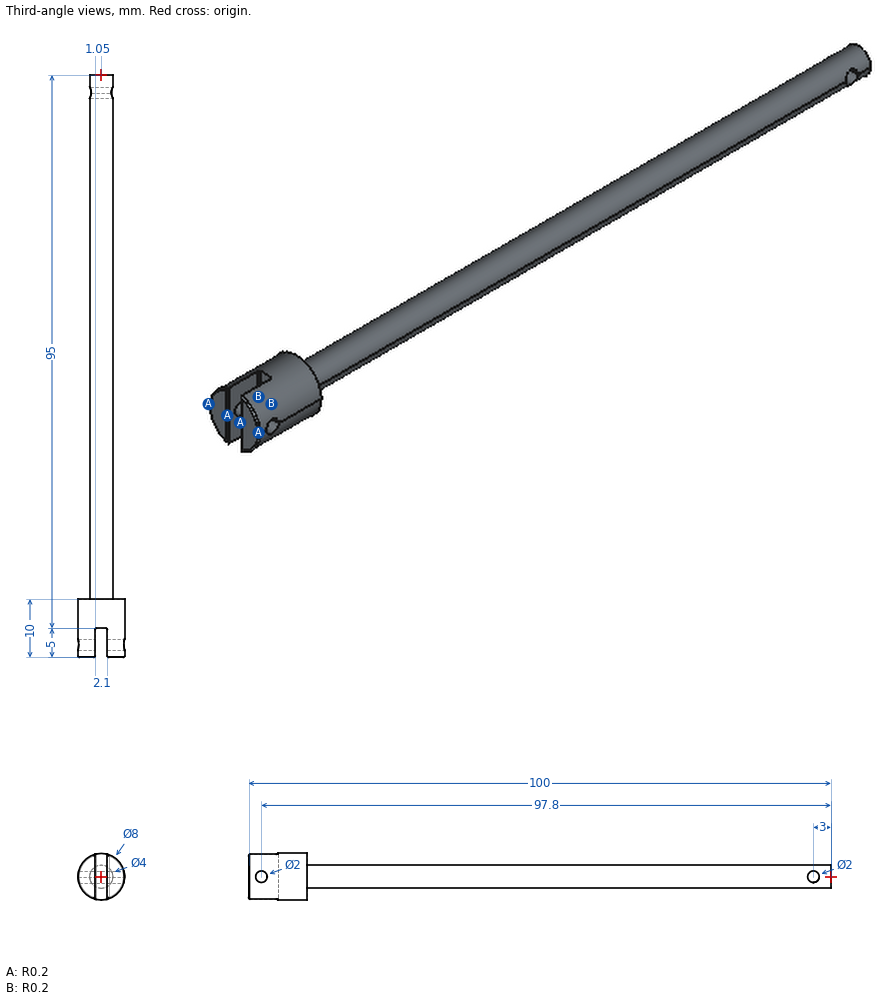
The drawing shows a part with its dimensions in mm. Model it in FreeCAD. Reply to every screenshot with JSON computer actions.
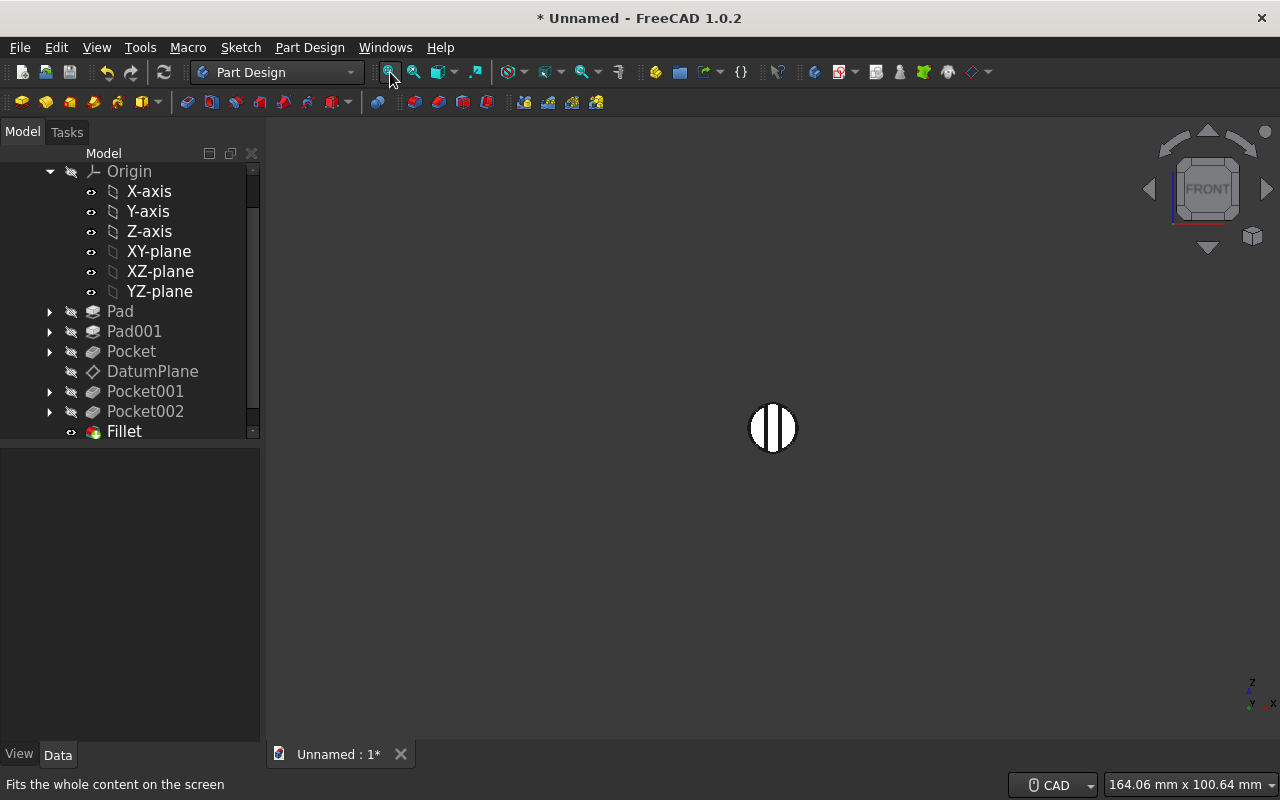
{"action": "left_click", "coordinate": [390, 72]}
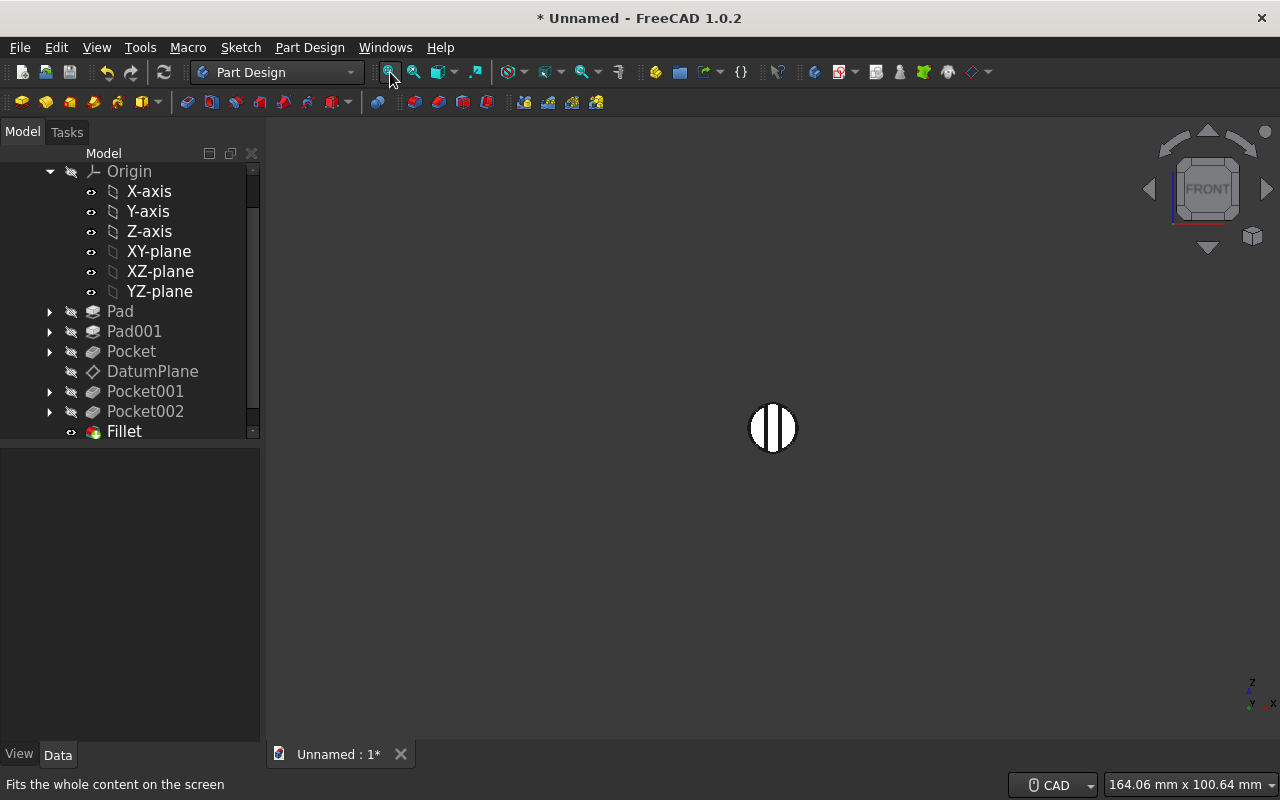
{"action": "key", "text": "3"}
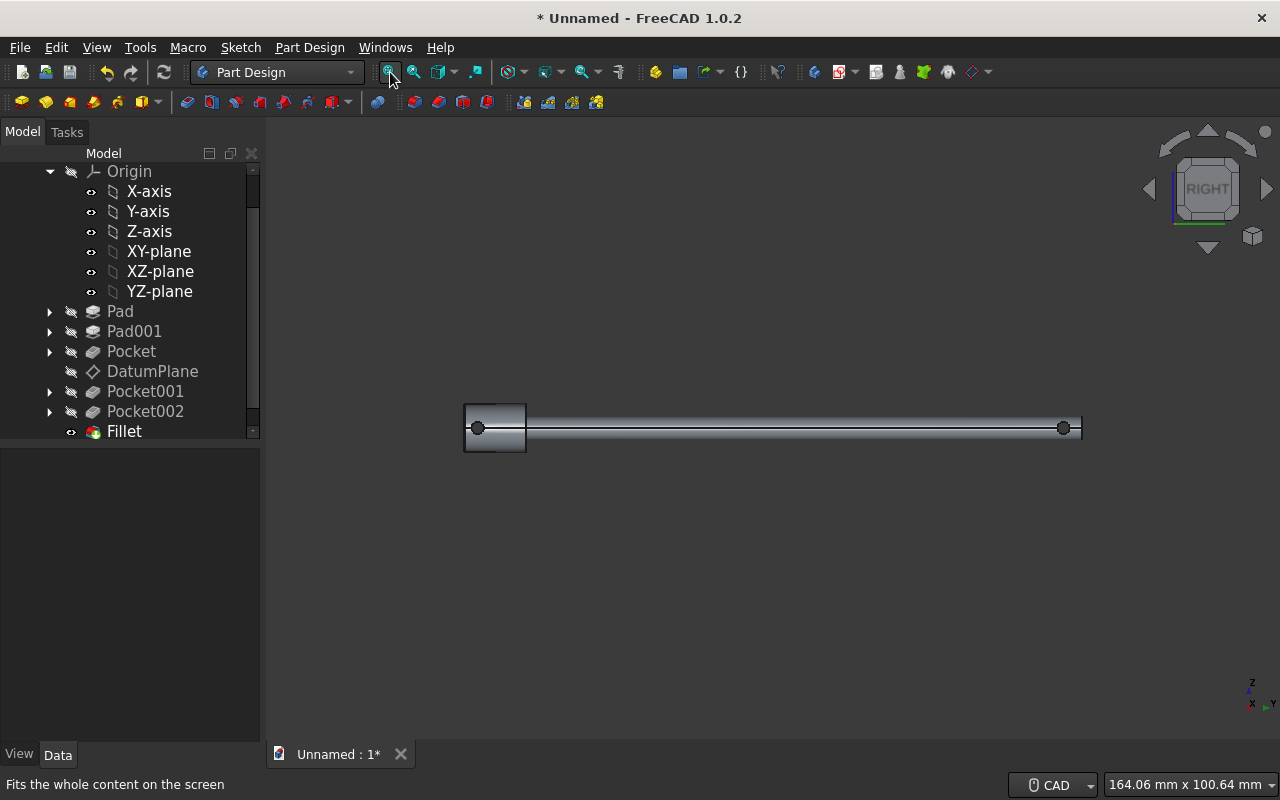
{"action": "key", "text": "5"}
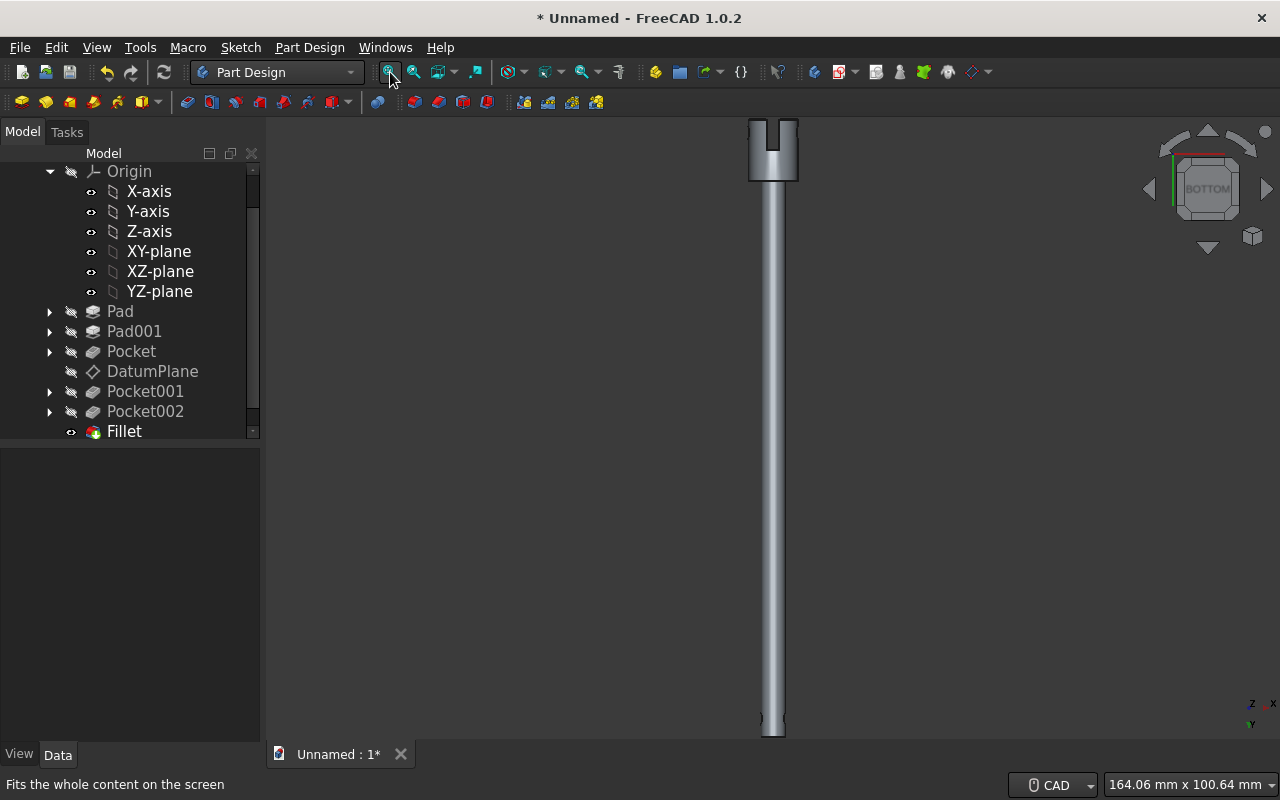
{"action": "key", "text": "4"}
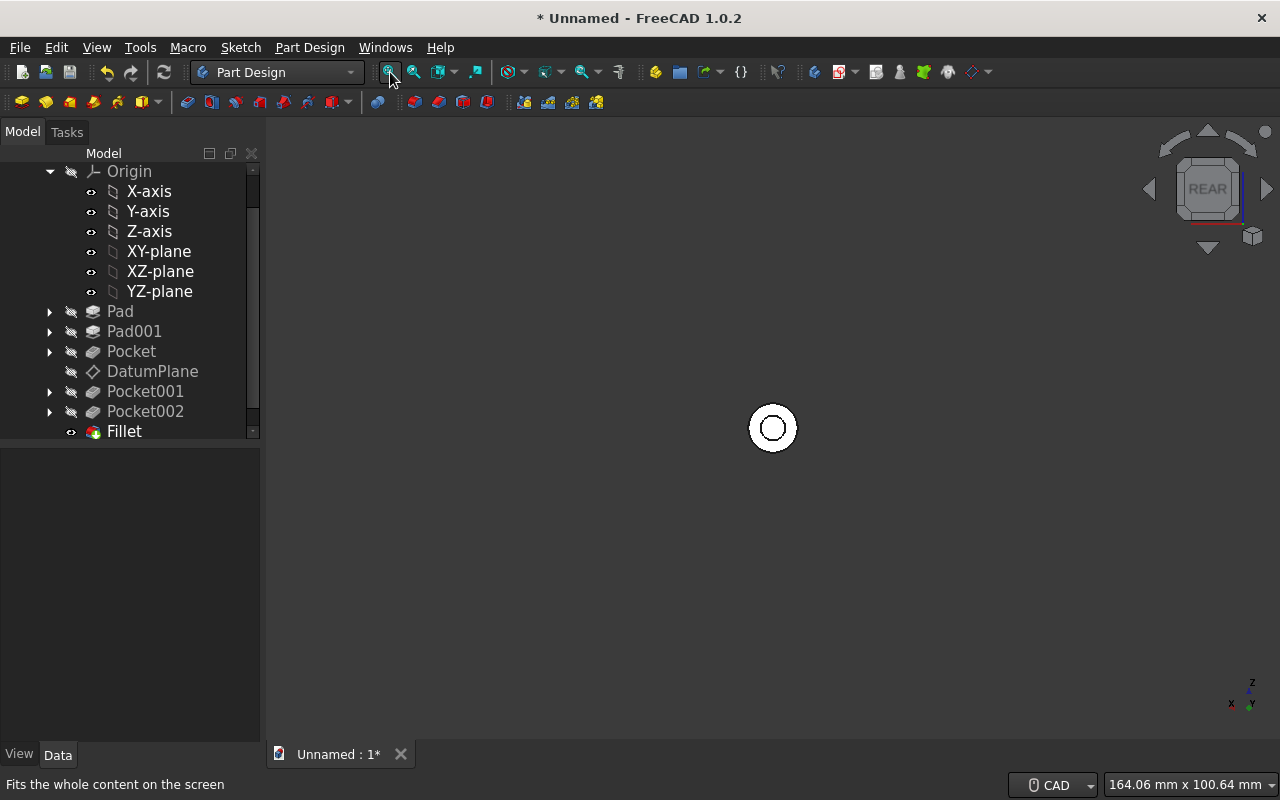
{"action": "left_click", "coordinate": [390, 72]}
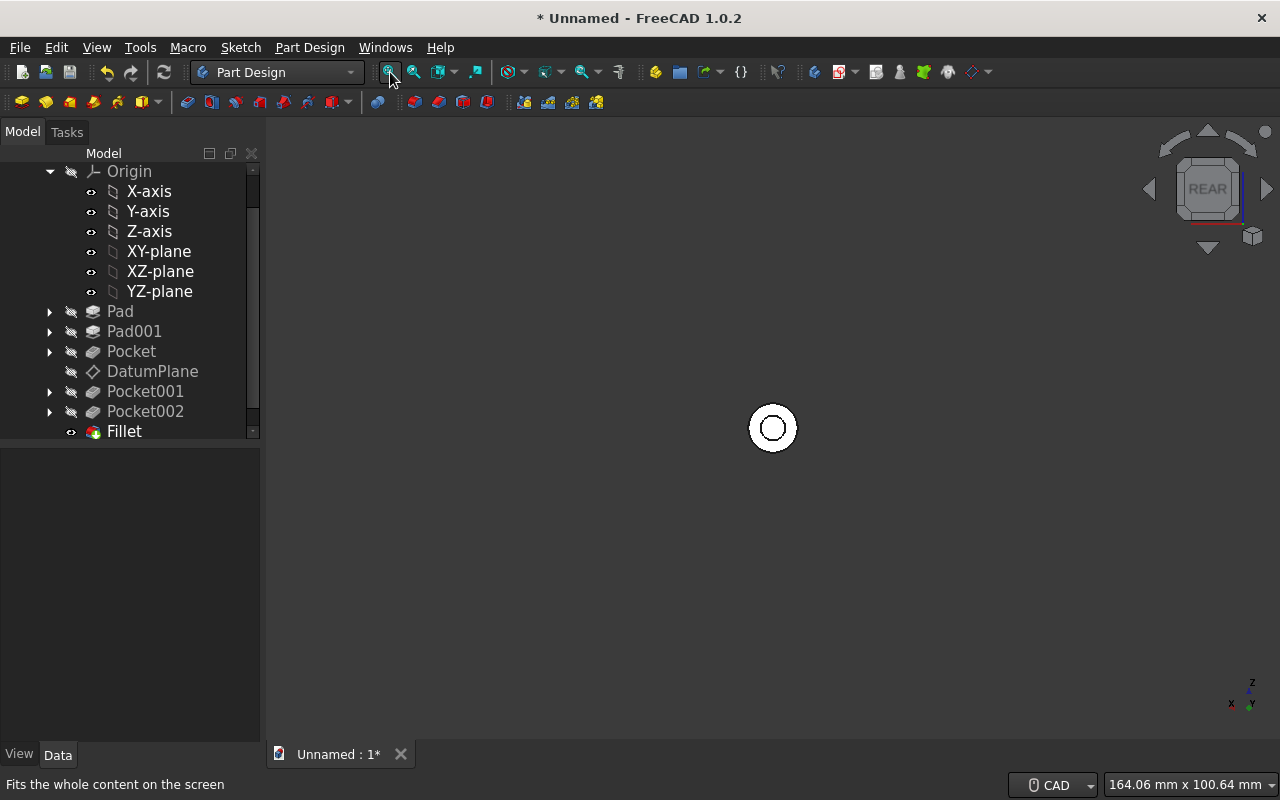
{"action": "key", "text": "6"}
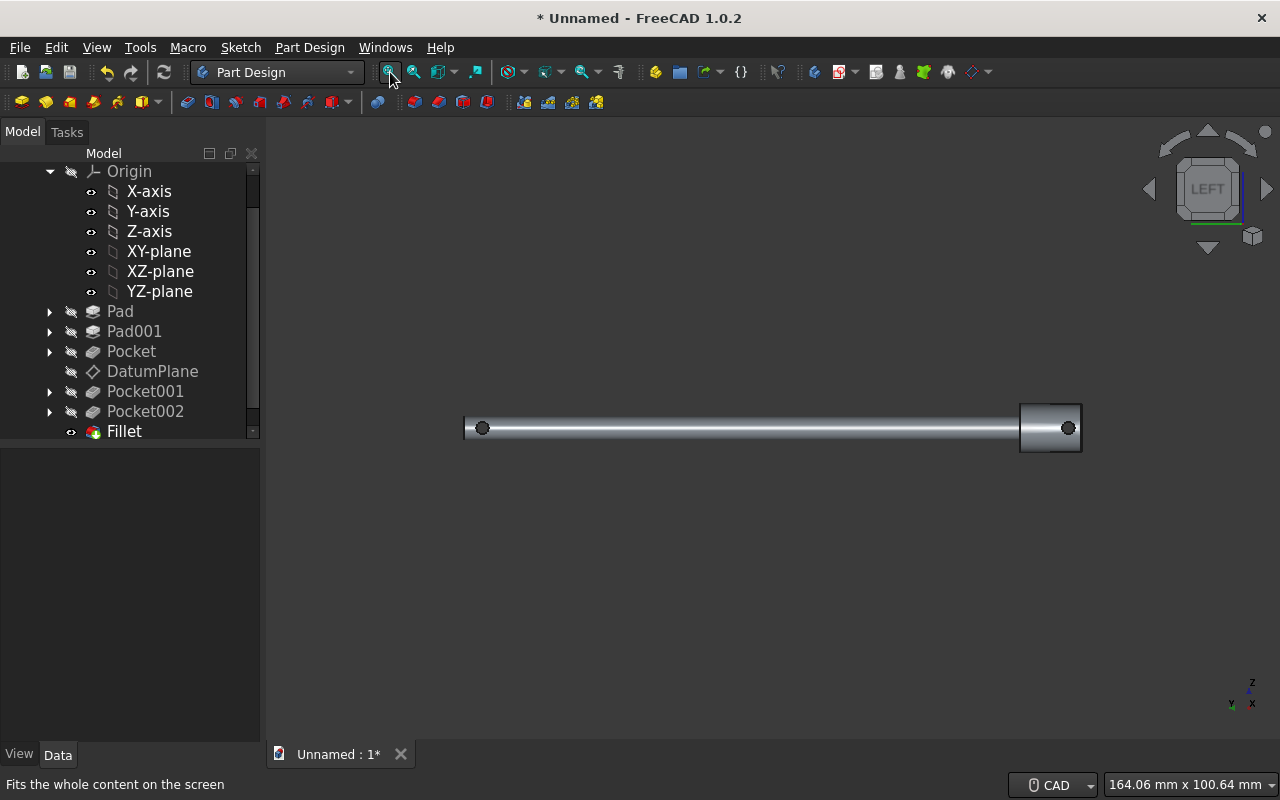
{"action": "key", "text": "v 3"}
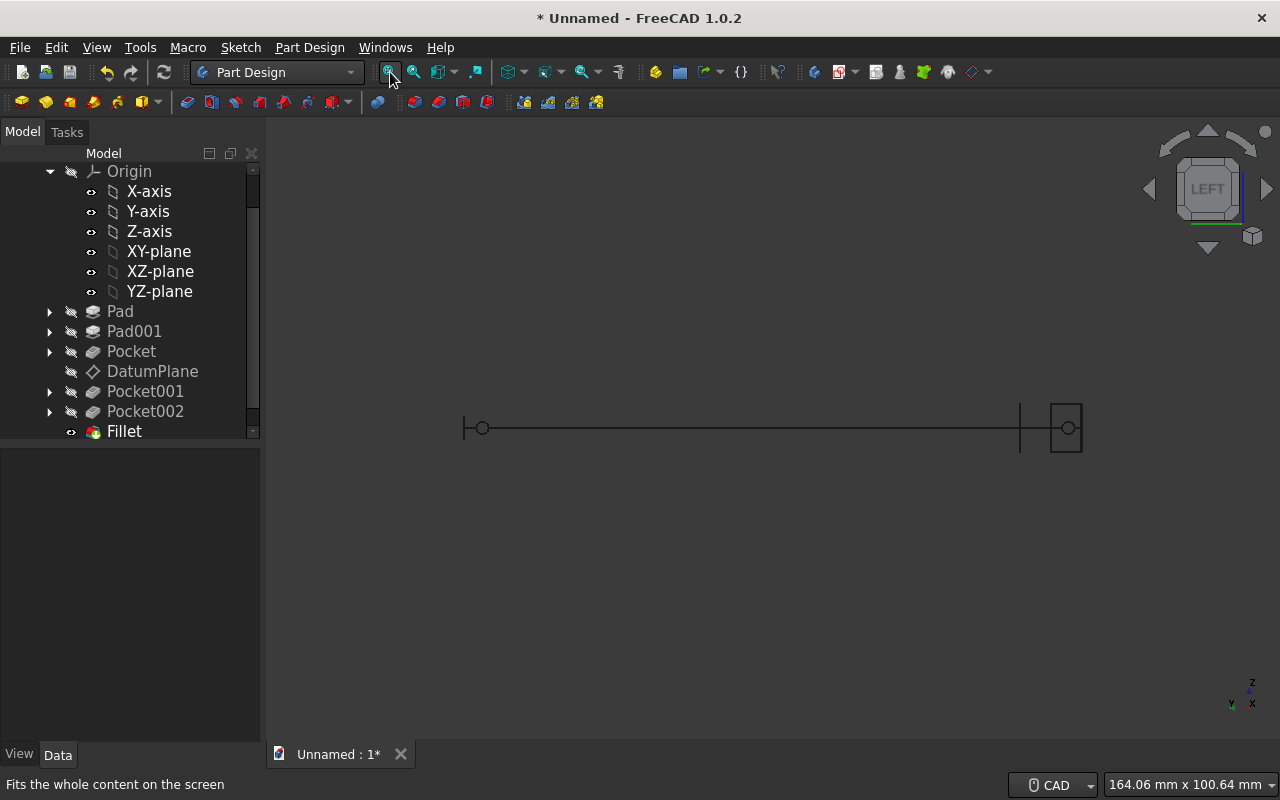
{"action": "key", "text": "0"}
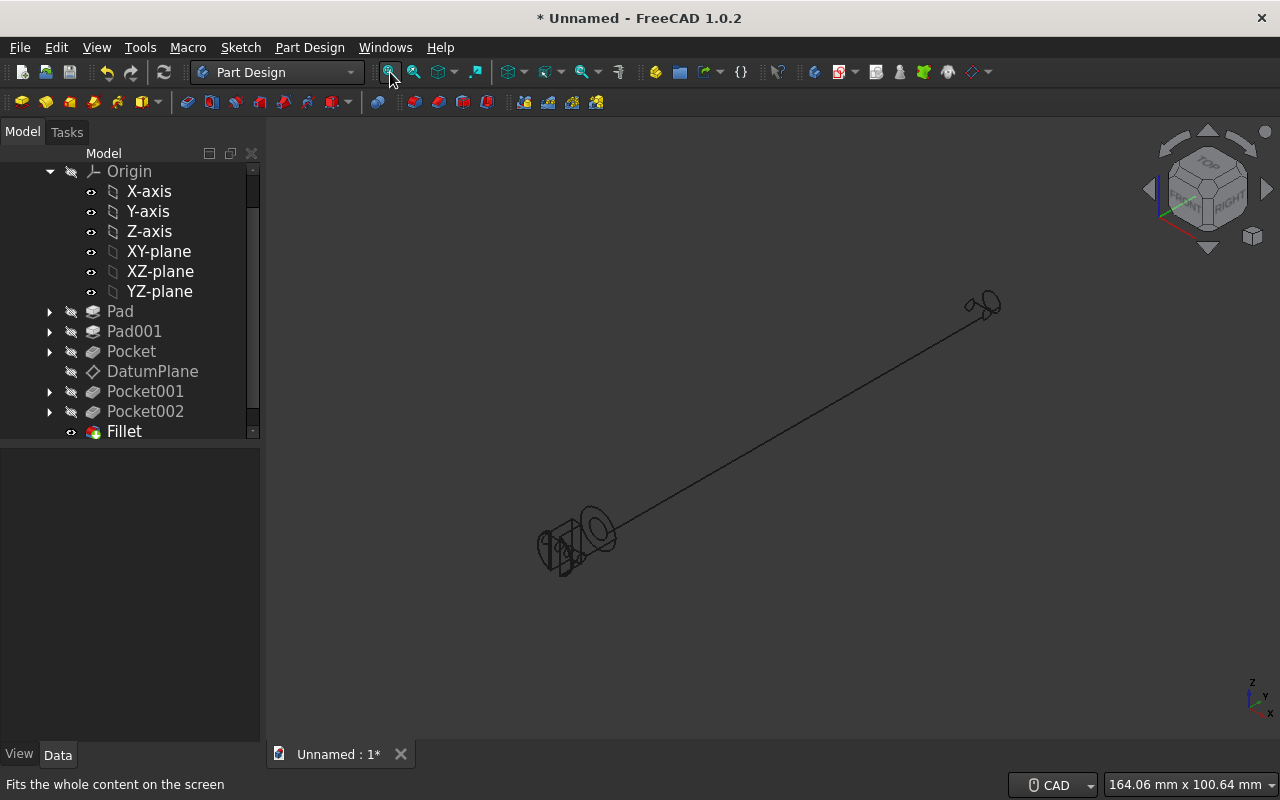
{"action": "left_click", "coordinate": [572, 538]}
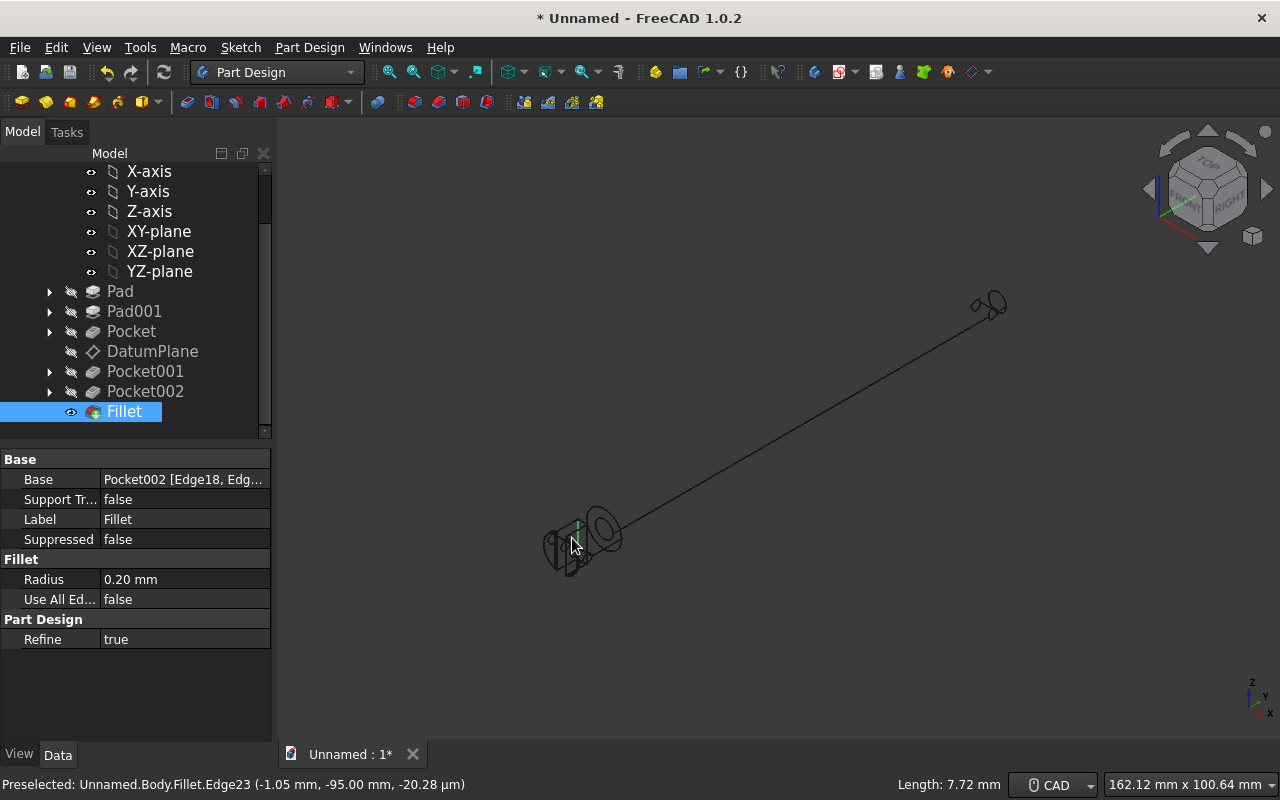
{"action": "left_click", "coordinate": [587, 543], "text": "ctrl"}